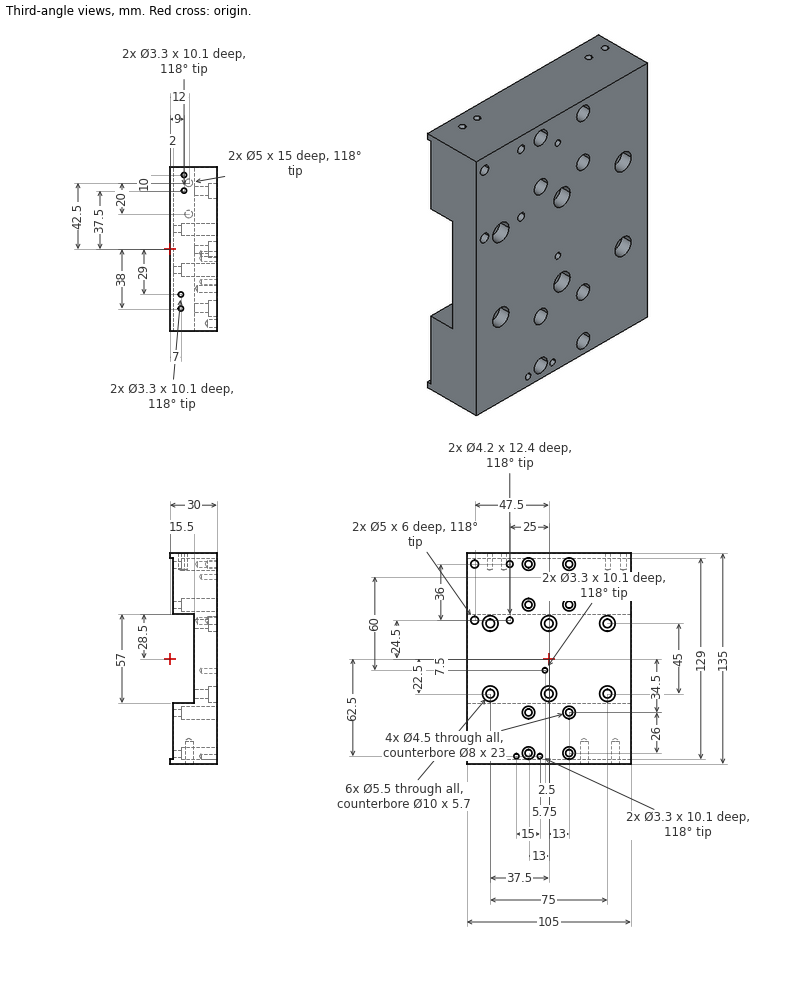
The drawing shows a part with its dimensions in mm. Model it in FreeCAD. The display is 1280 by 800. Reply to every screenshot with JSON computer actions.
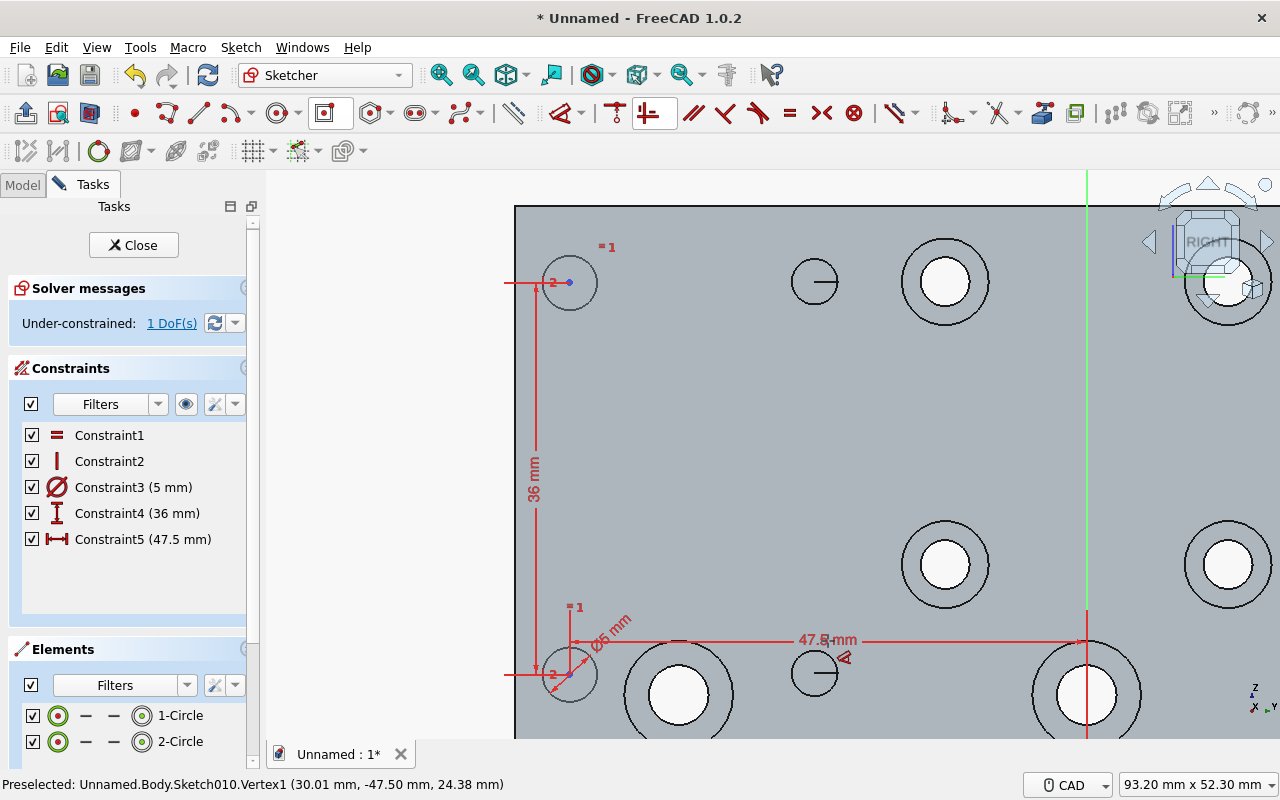
{"action": "left_click", "coordinate": [570, 675]}
{"action": "left_click", "coordinate": [536, 701]}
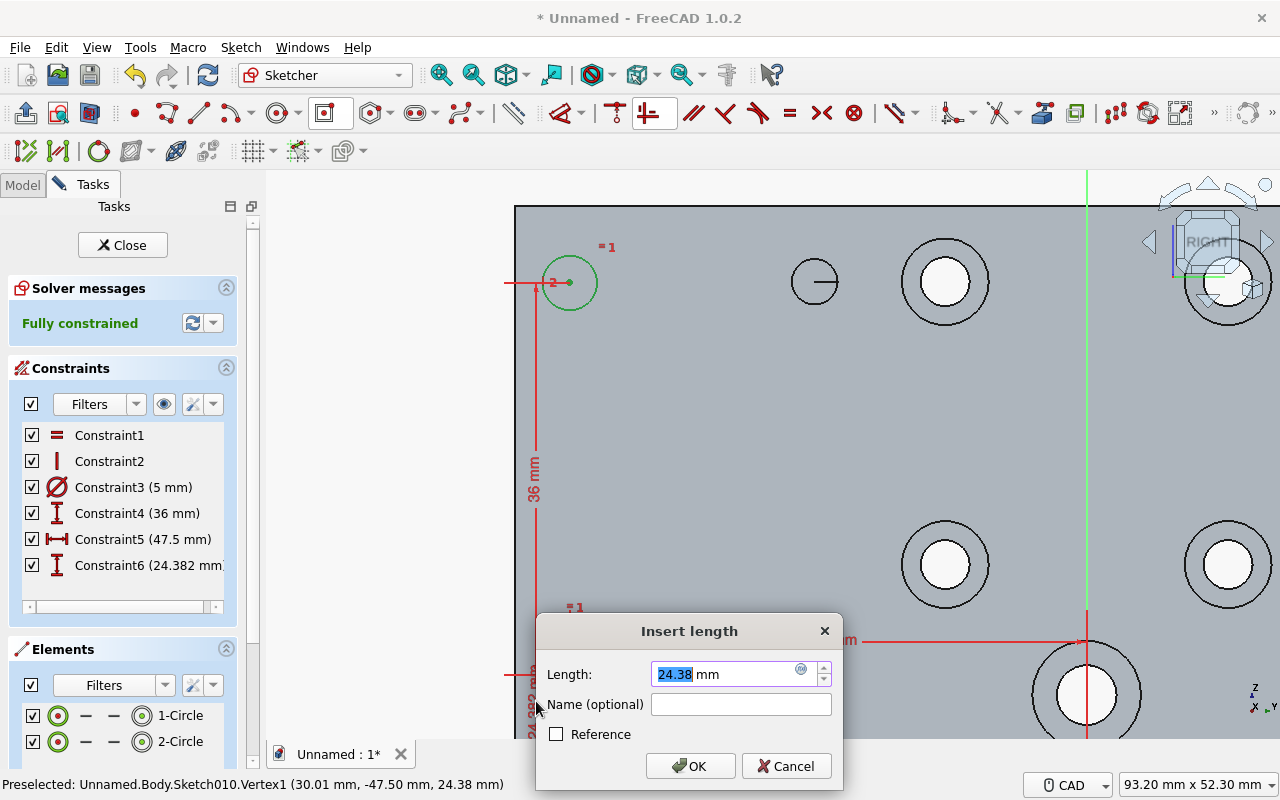
{"action": "type", "text": "24.5"}
{"action": "key", "text": "Return"}
{"action": "key", "text": "Escape"}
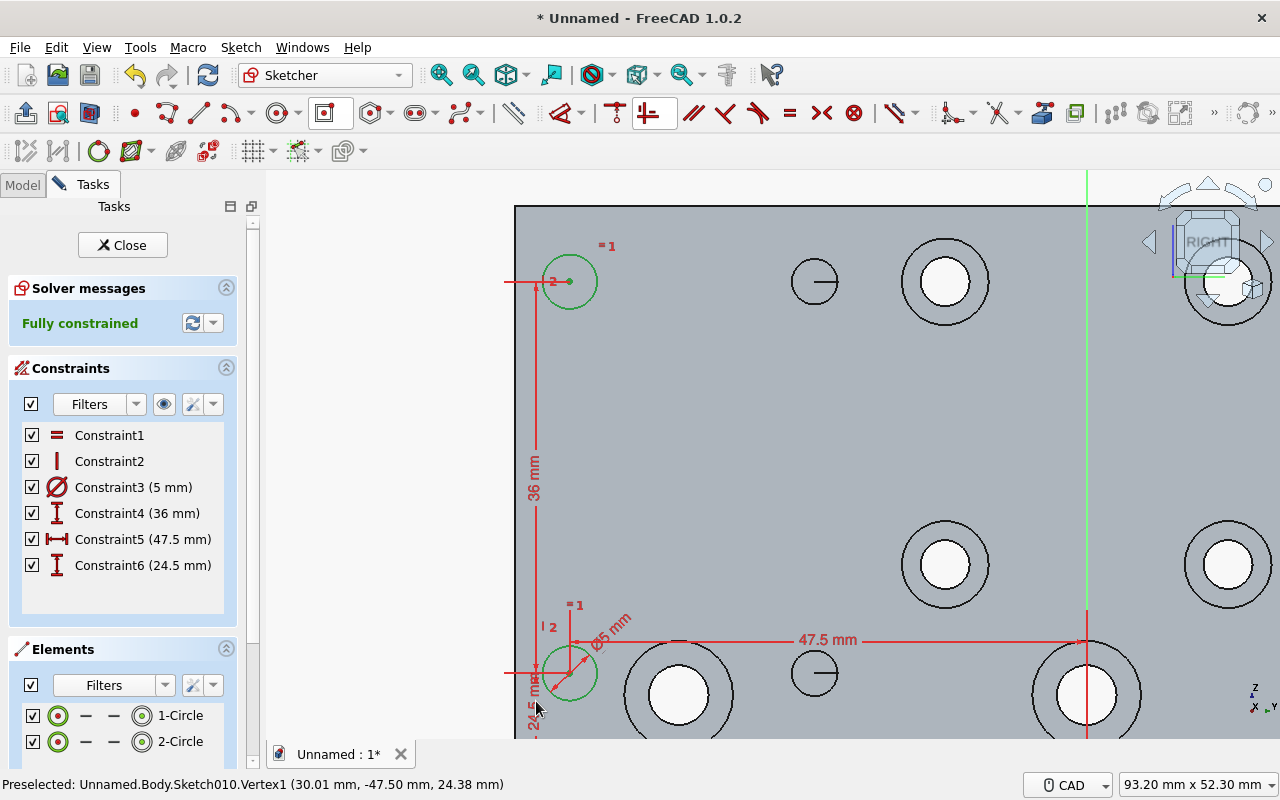
{"action": "left_click", "coordinate": [123, 245]}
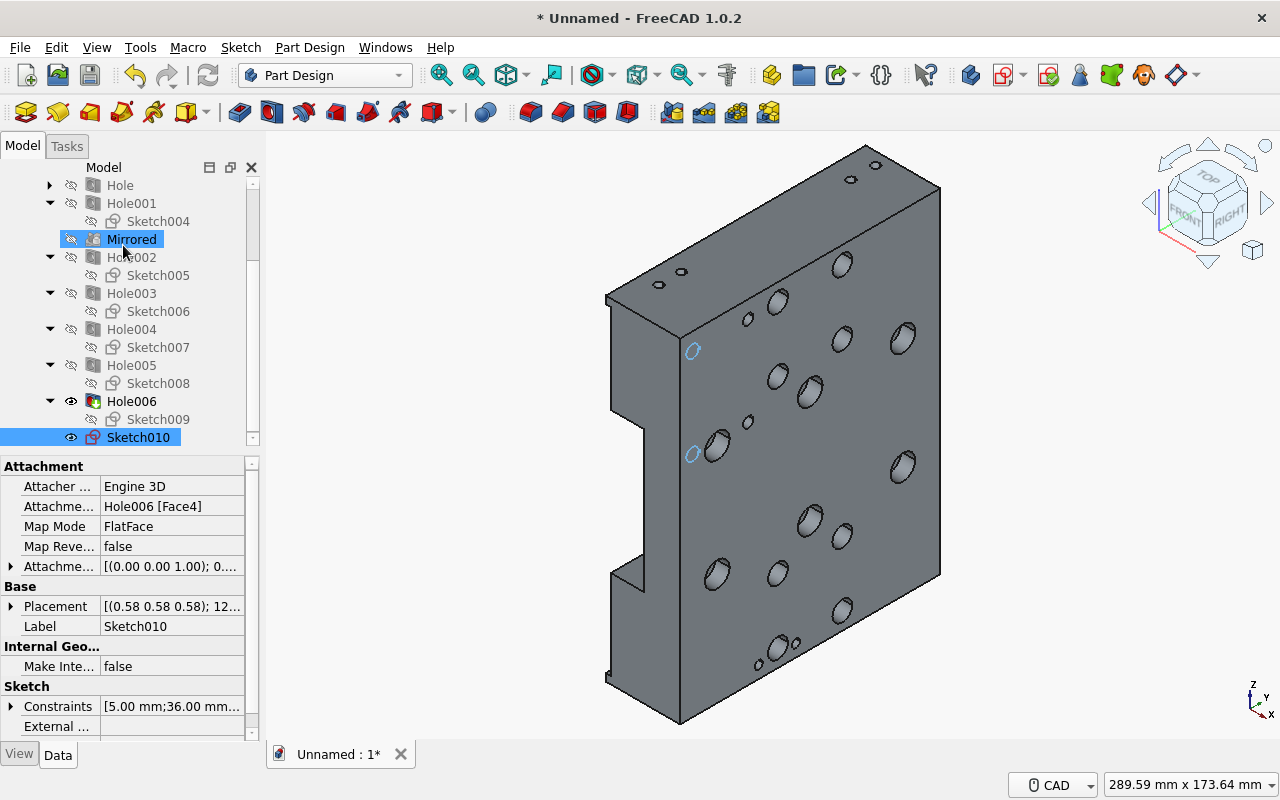
{"action": "left_click", "coordinate": [272, 112]}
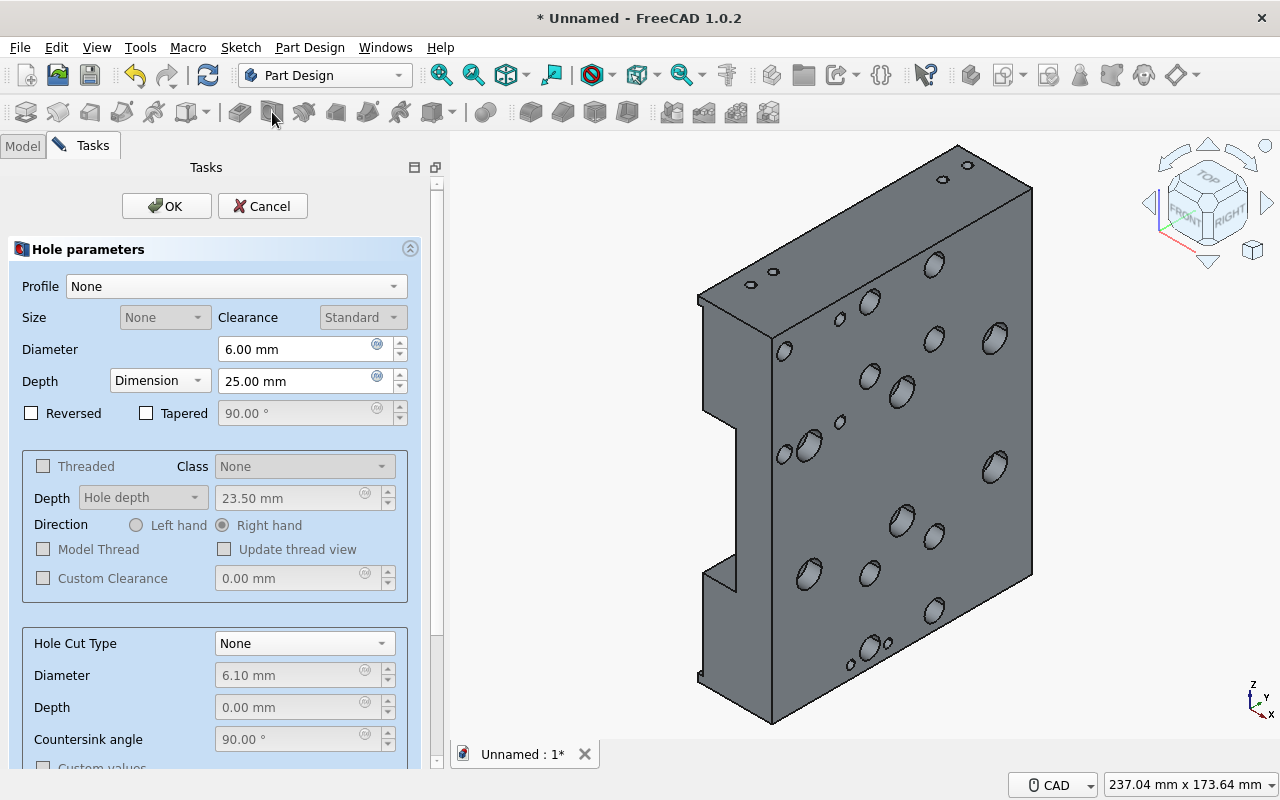
{"action": "triple_click", "coordinate": [305, 349]}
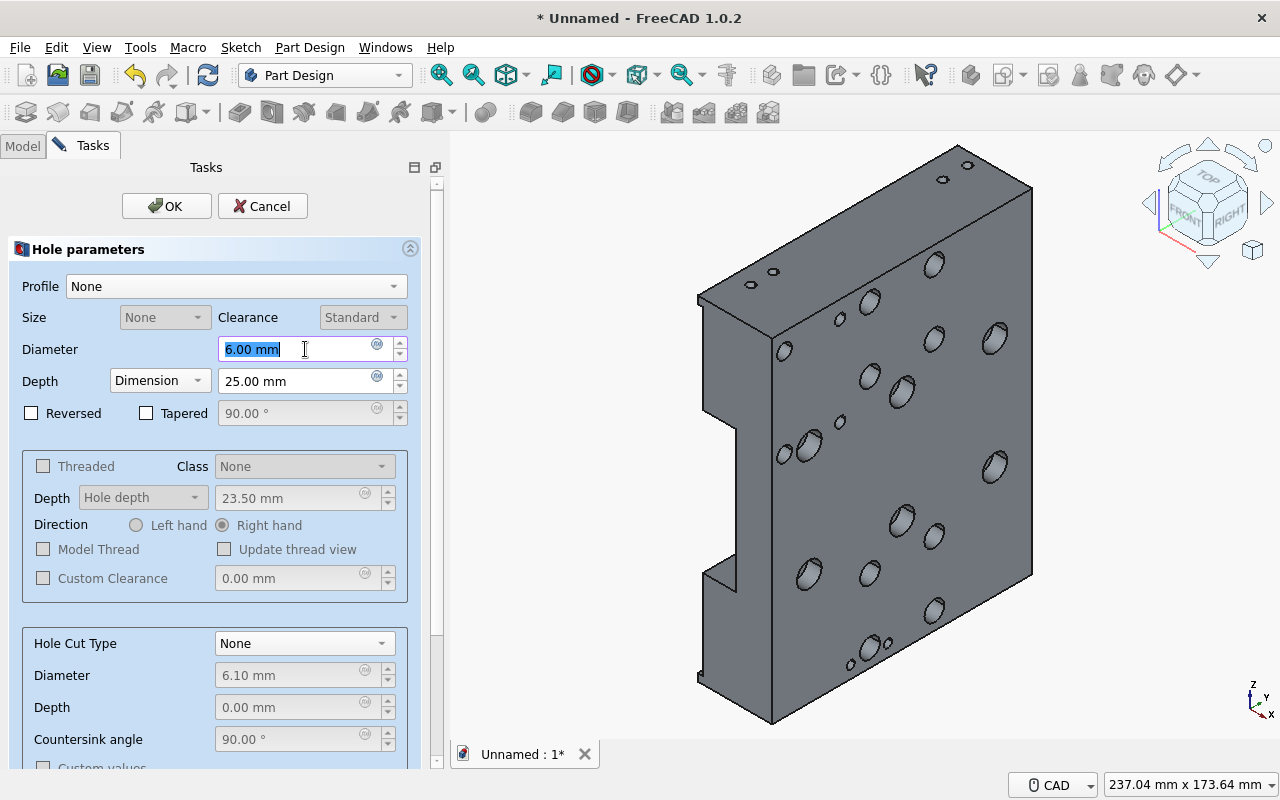
{"action": "type", "text": "5"}
{"action": "key", "text": "Tab"}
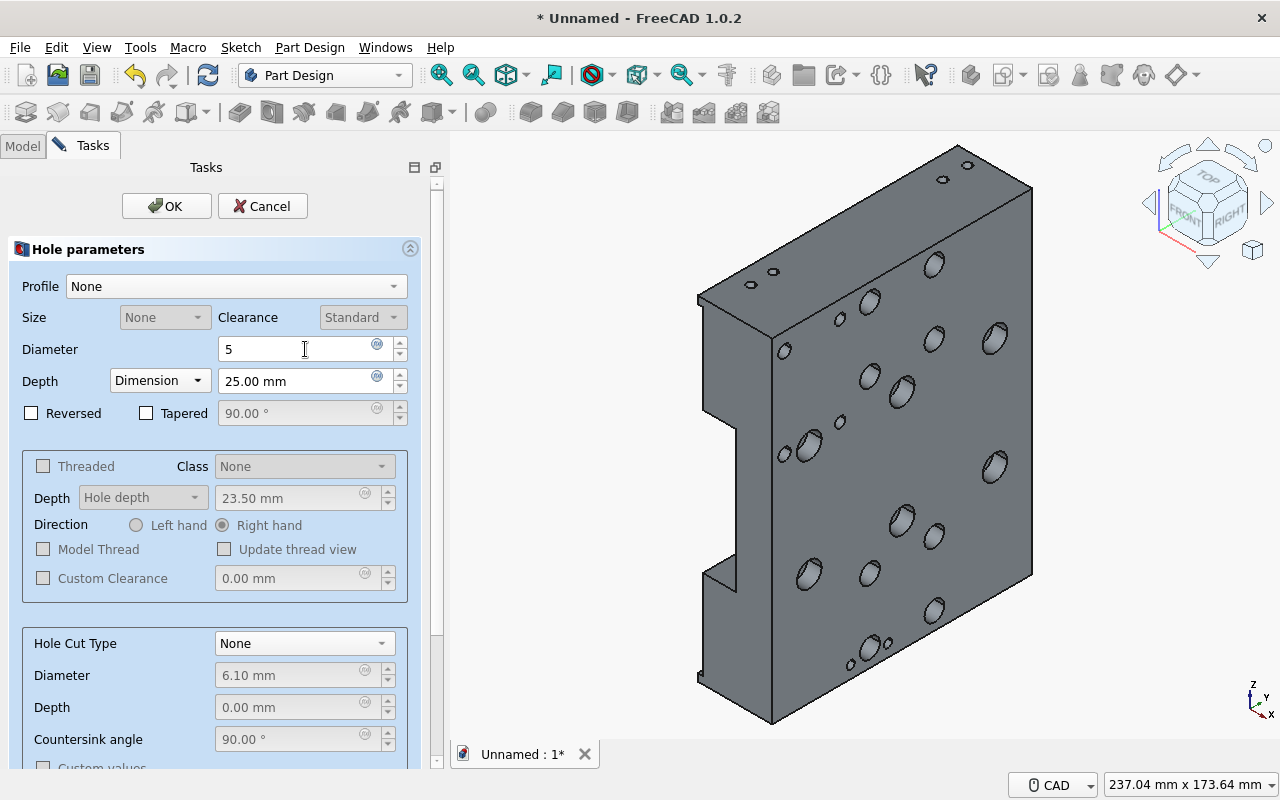
{"action": "triple_click", "coordinate": [305, 381]}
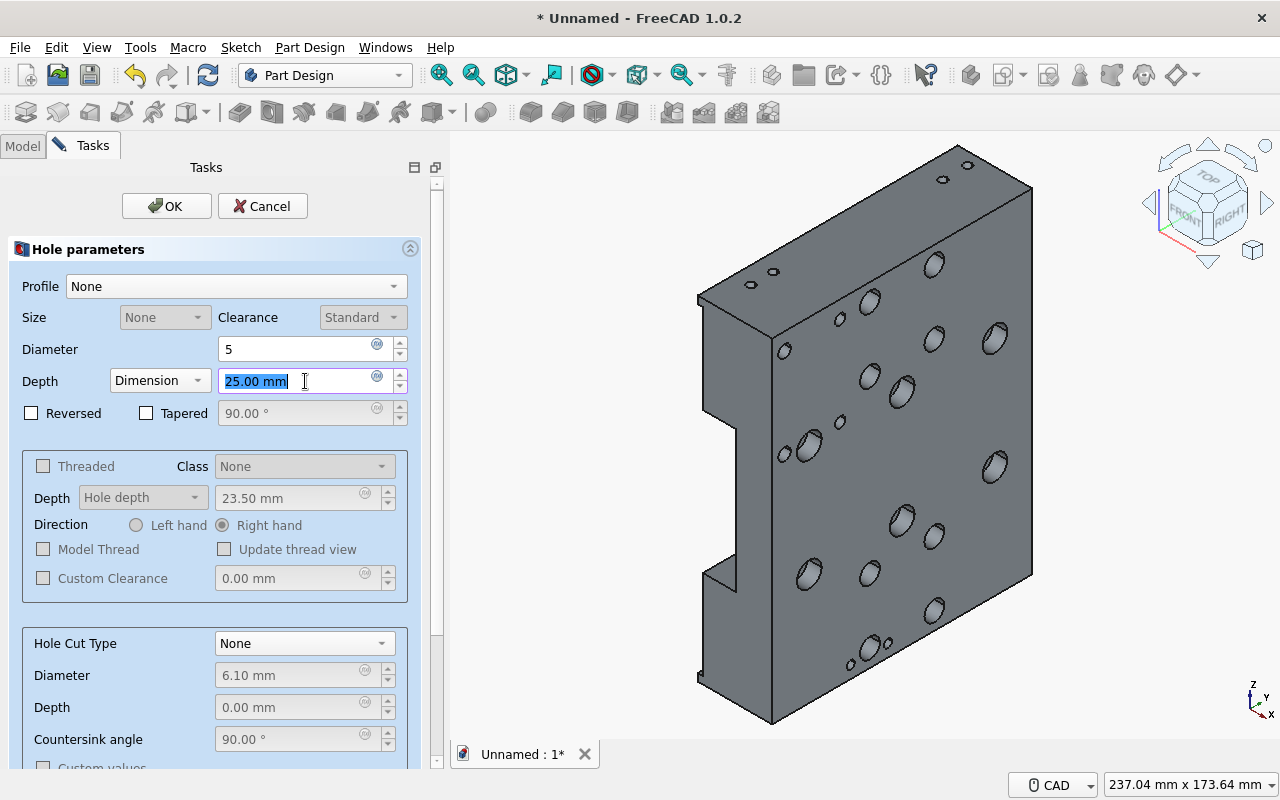
{"action": "type", "text": "6"}
{"action": "key", "text": "Tab"}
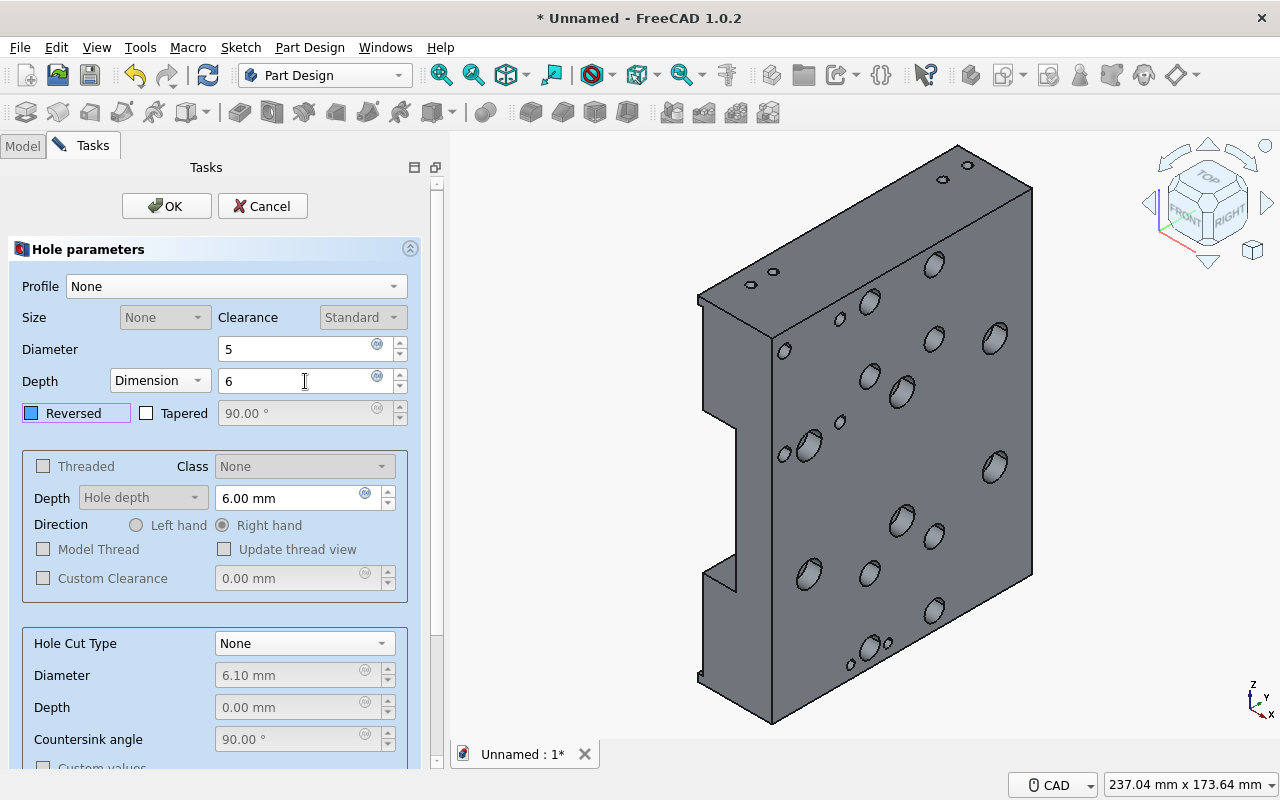
{"action": "left_click", "coordinate": [167, 206]}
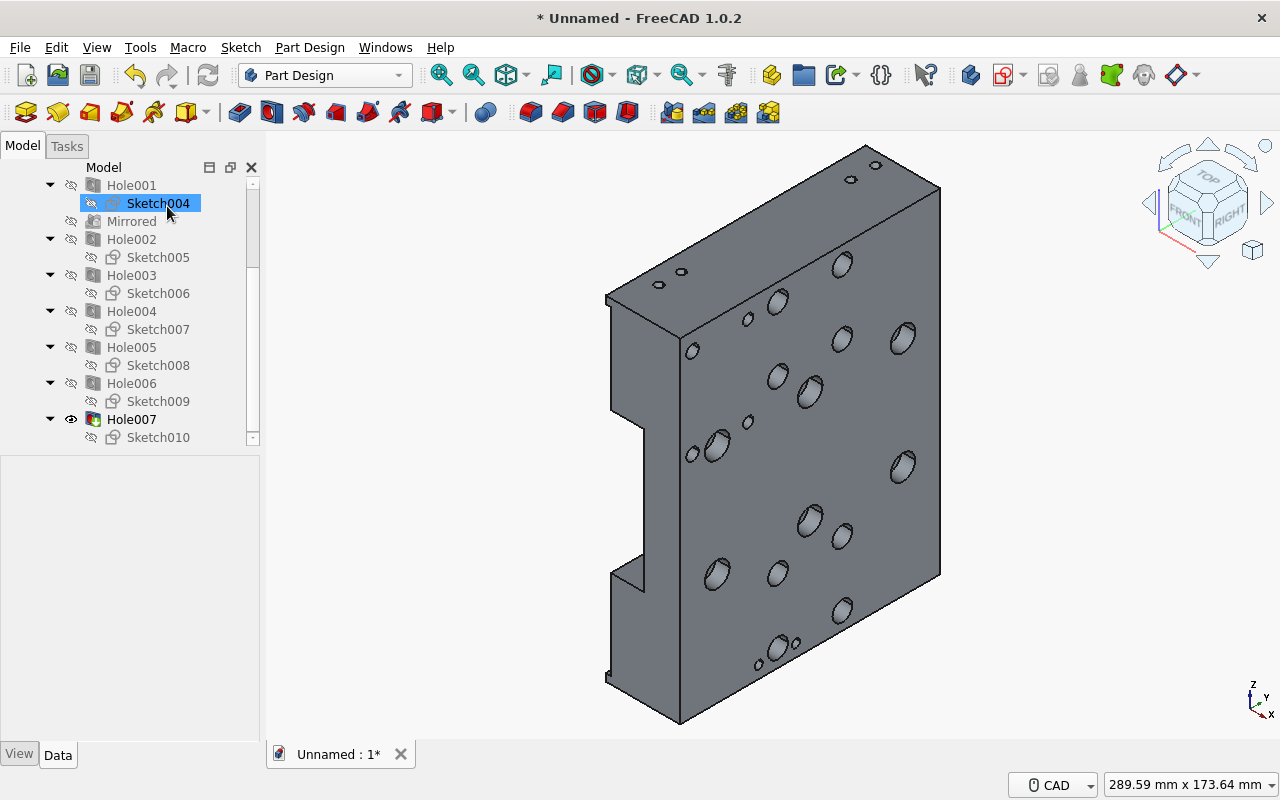
{"action": "left_click", "coordinate": [847, 434]}